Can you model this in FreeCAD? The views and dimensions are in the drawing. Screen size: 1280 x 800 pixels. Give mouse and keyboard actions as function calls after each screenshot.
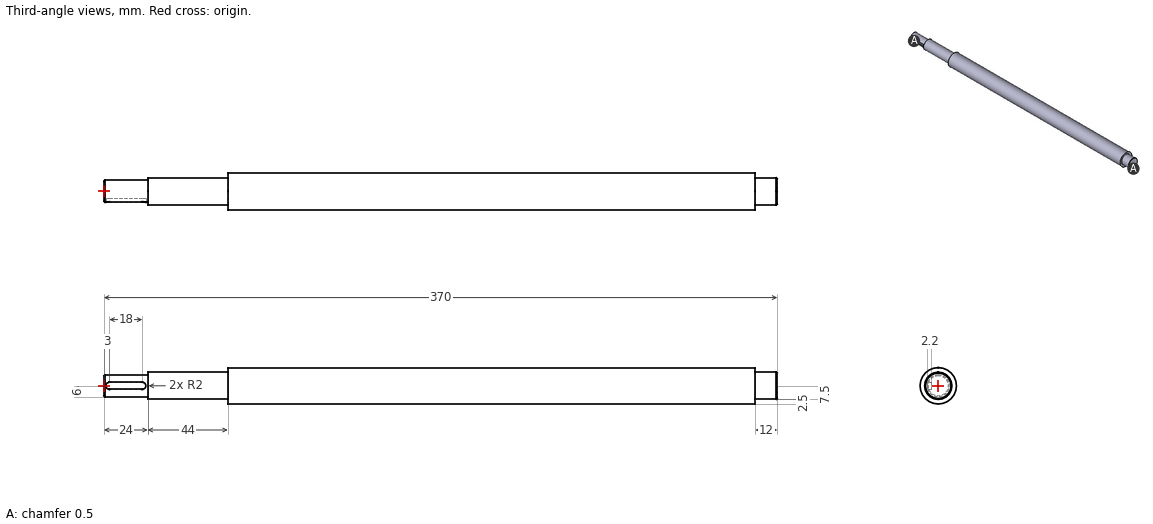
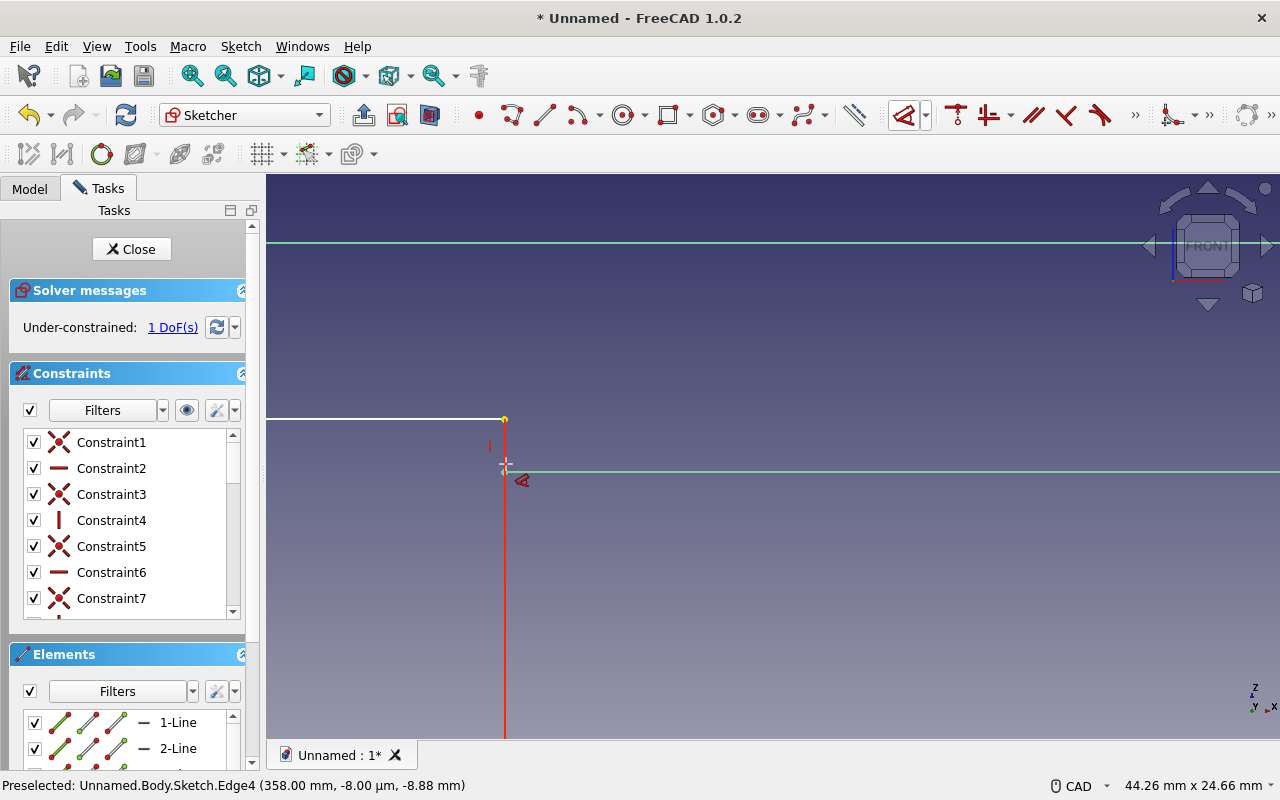
click(505, 456)
click(471, 446)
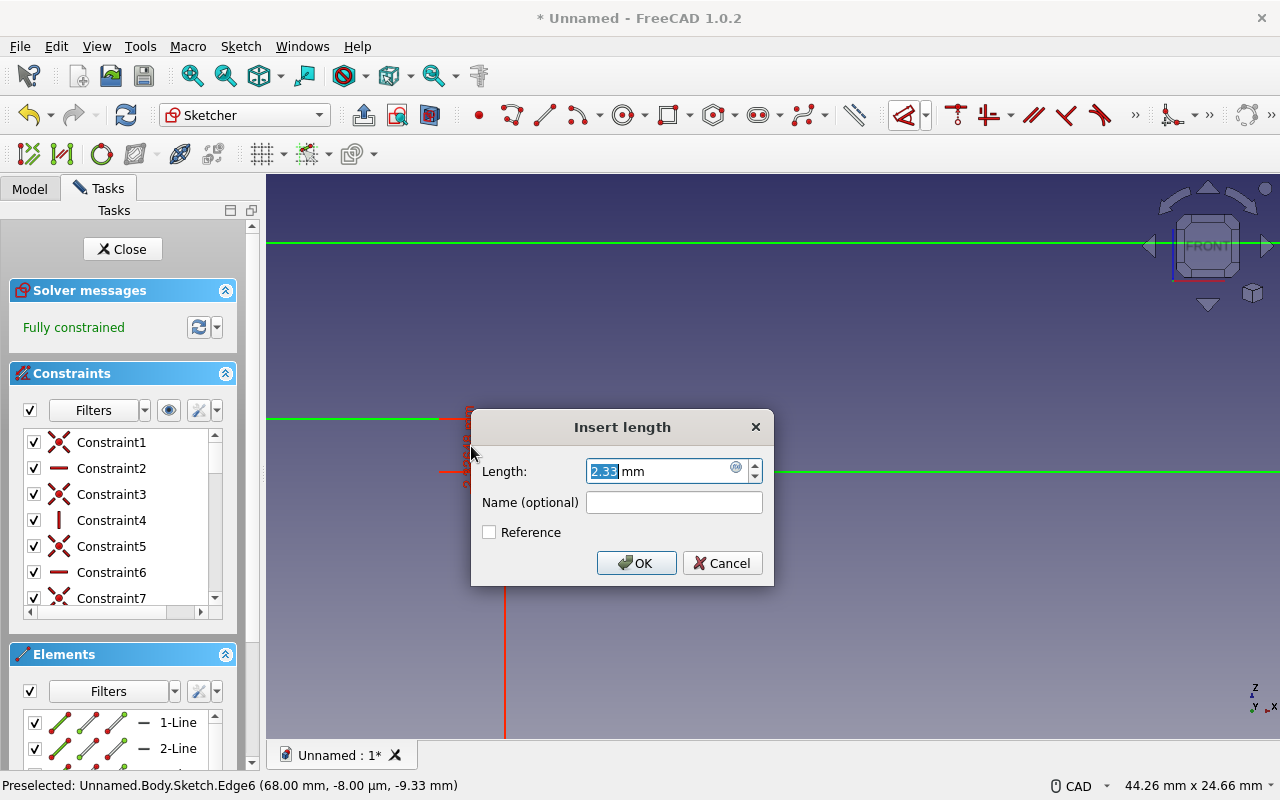
text(2.5)
key(Return)
key(Escape)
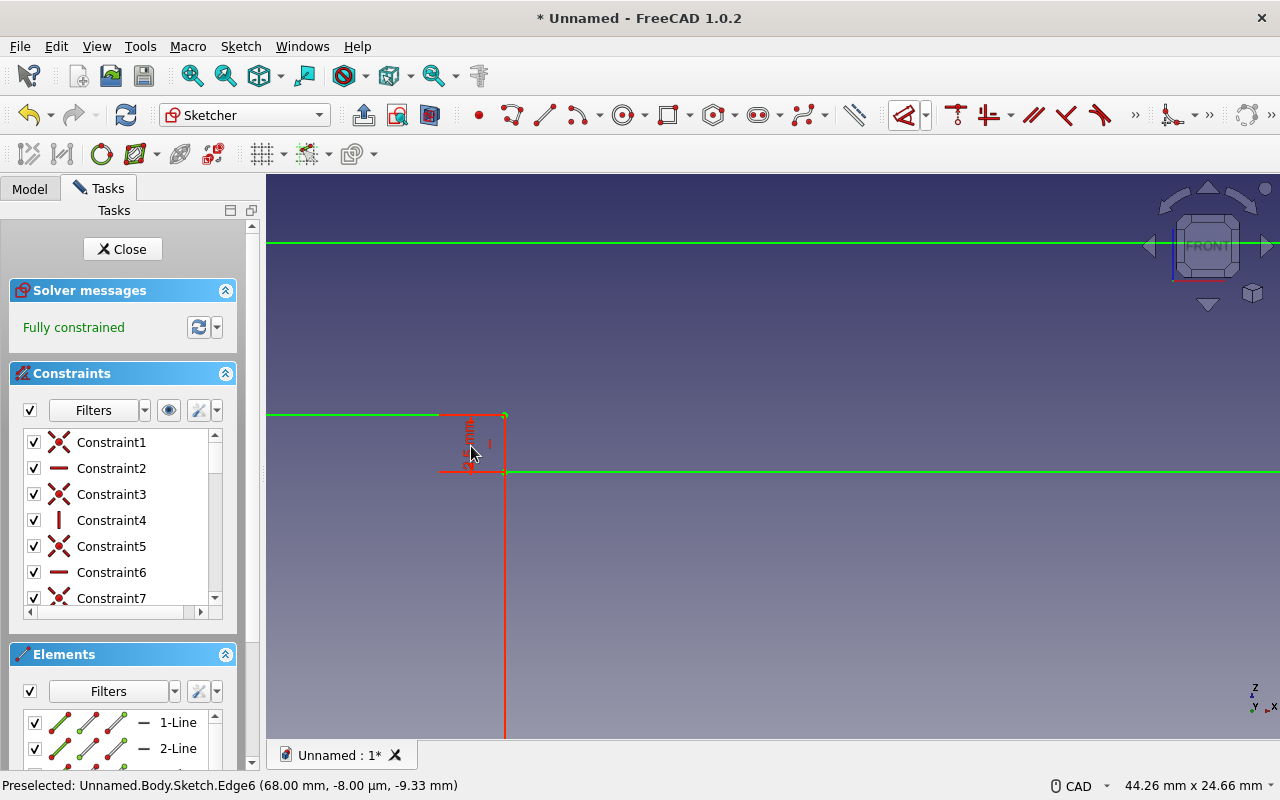
click(123, 249)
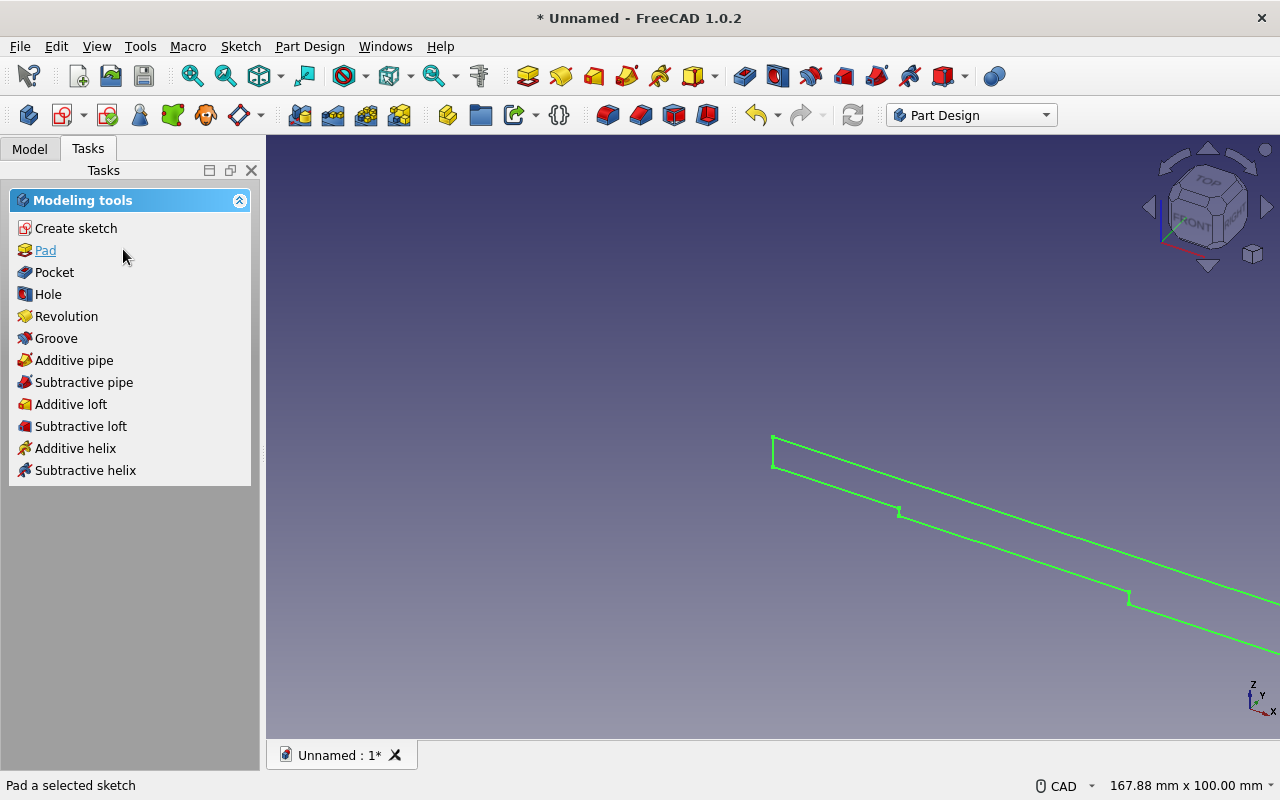
click(561, 76)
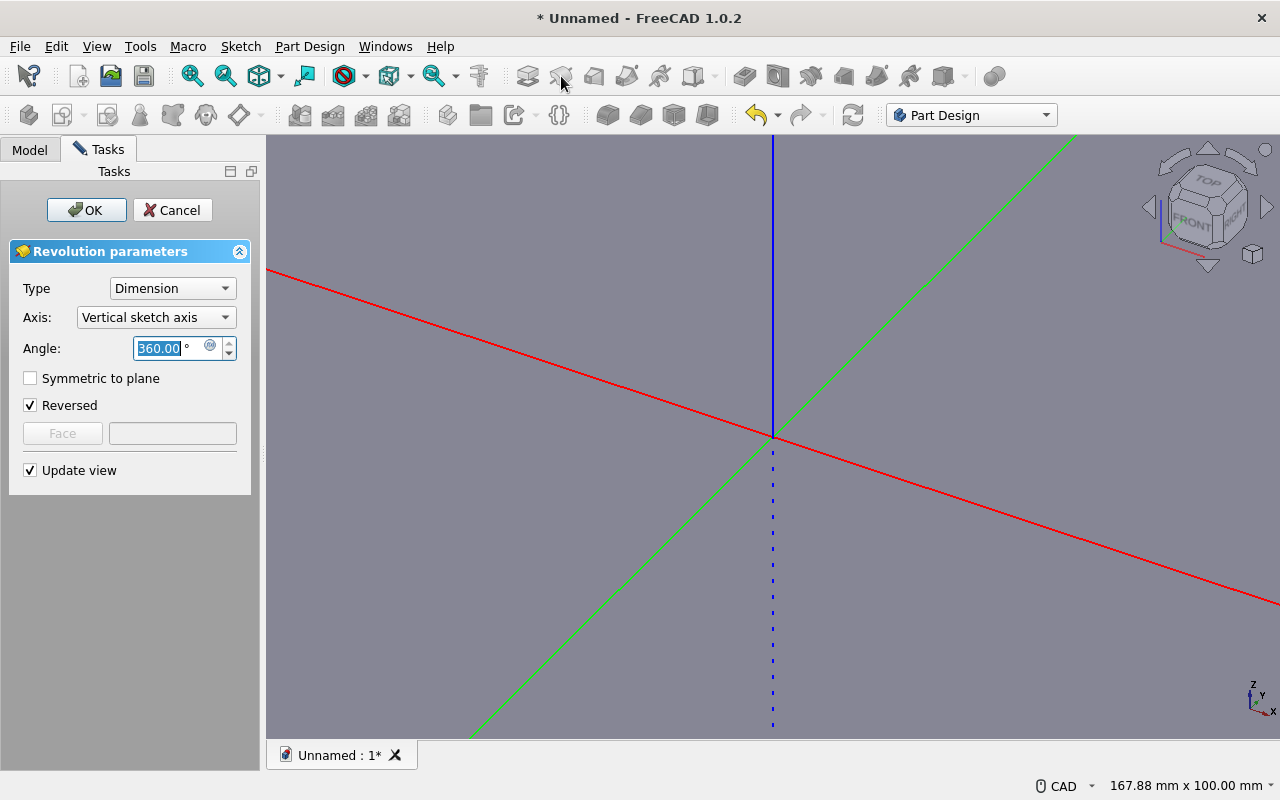
click(157, 318)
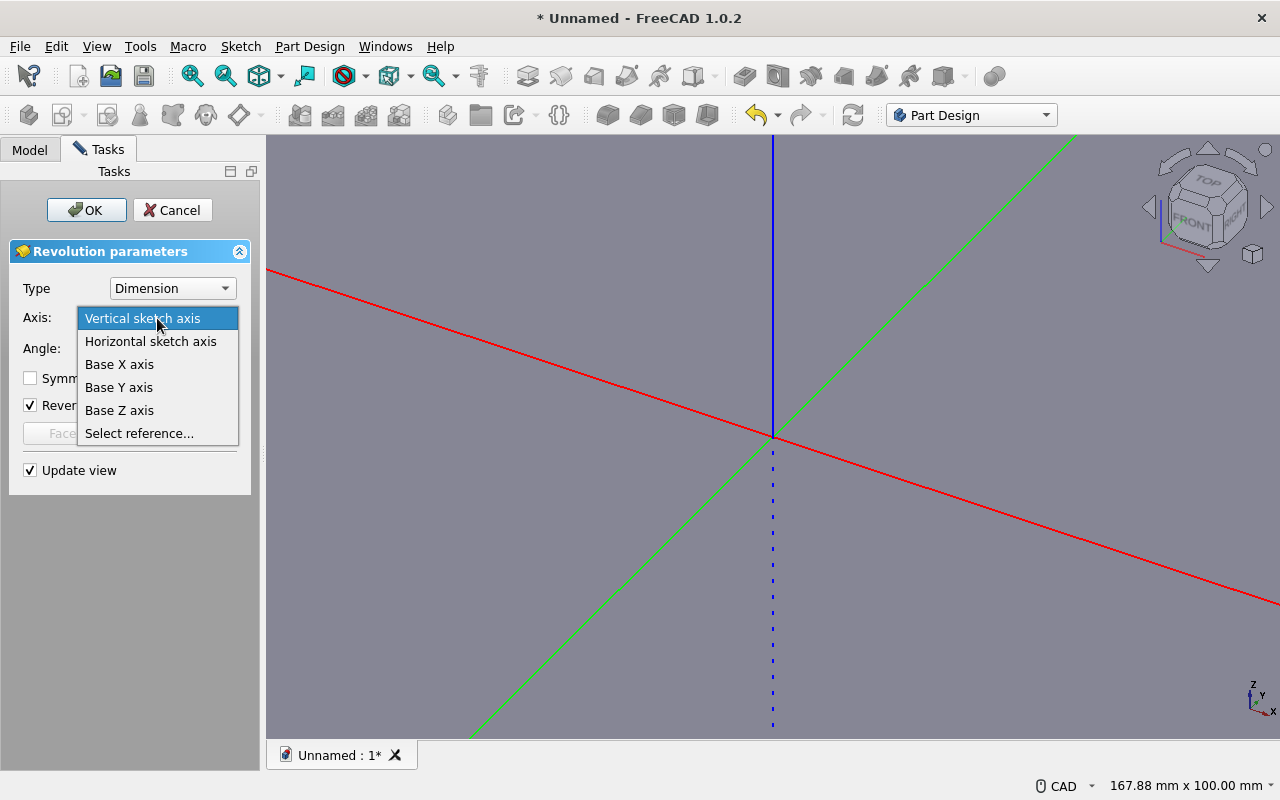
click(156, 342)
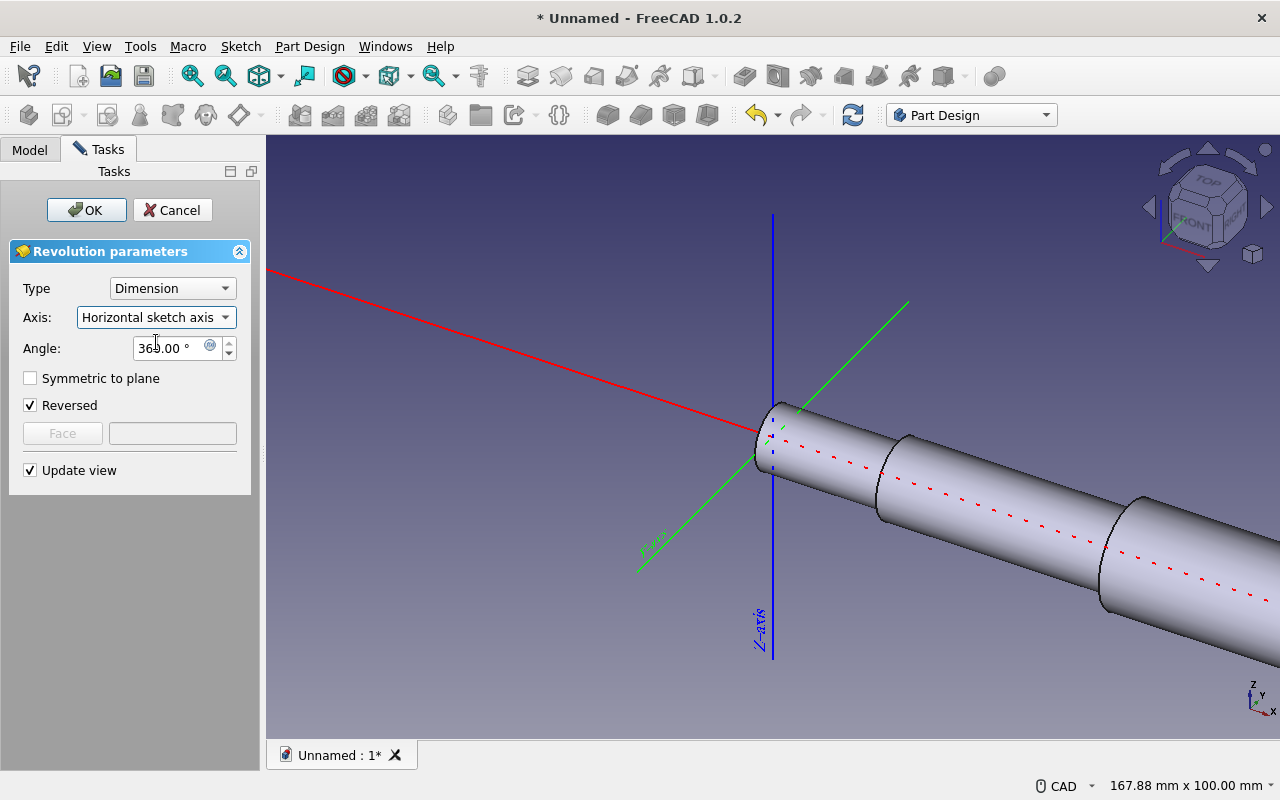
click(87, 210)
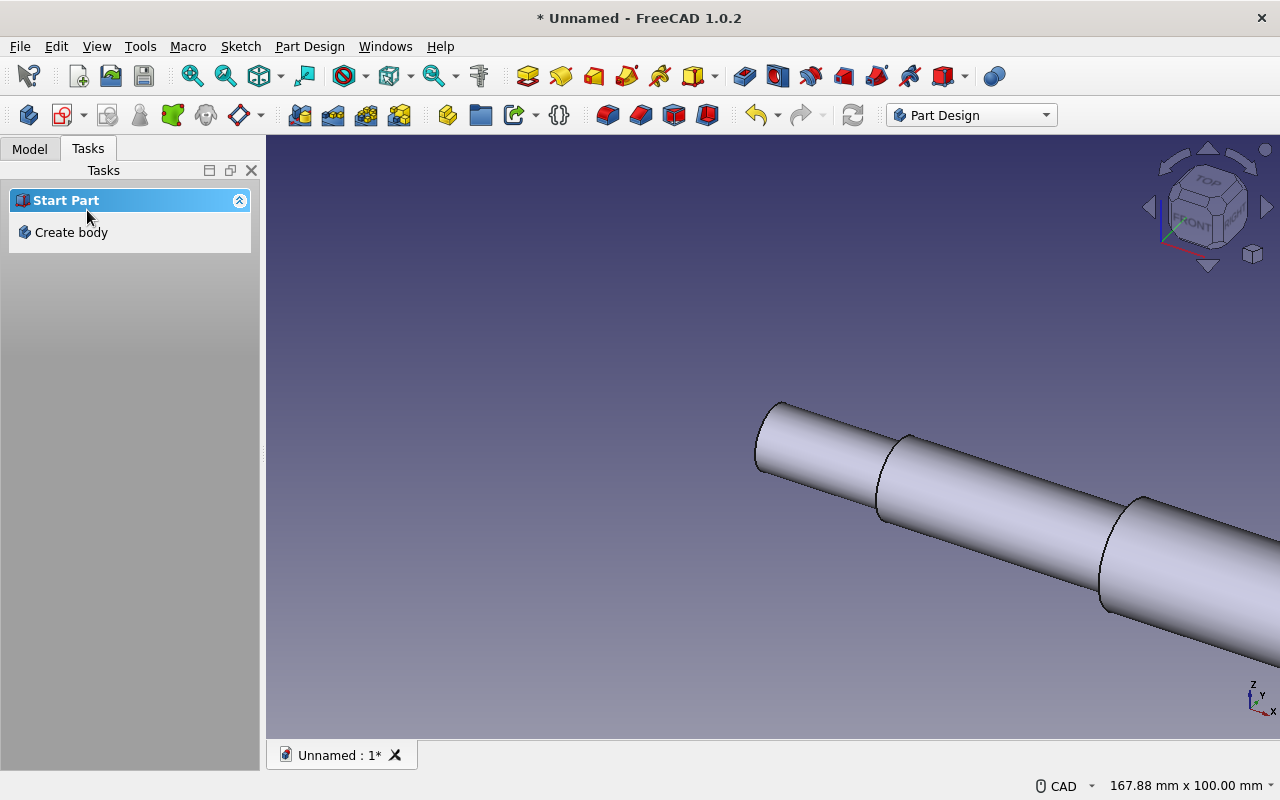
key(v)
key(f)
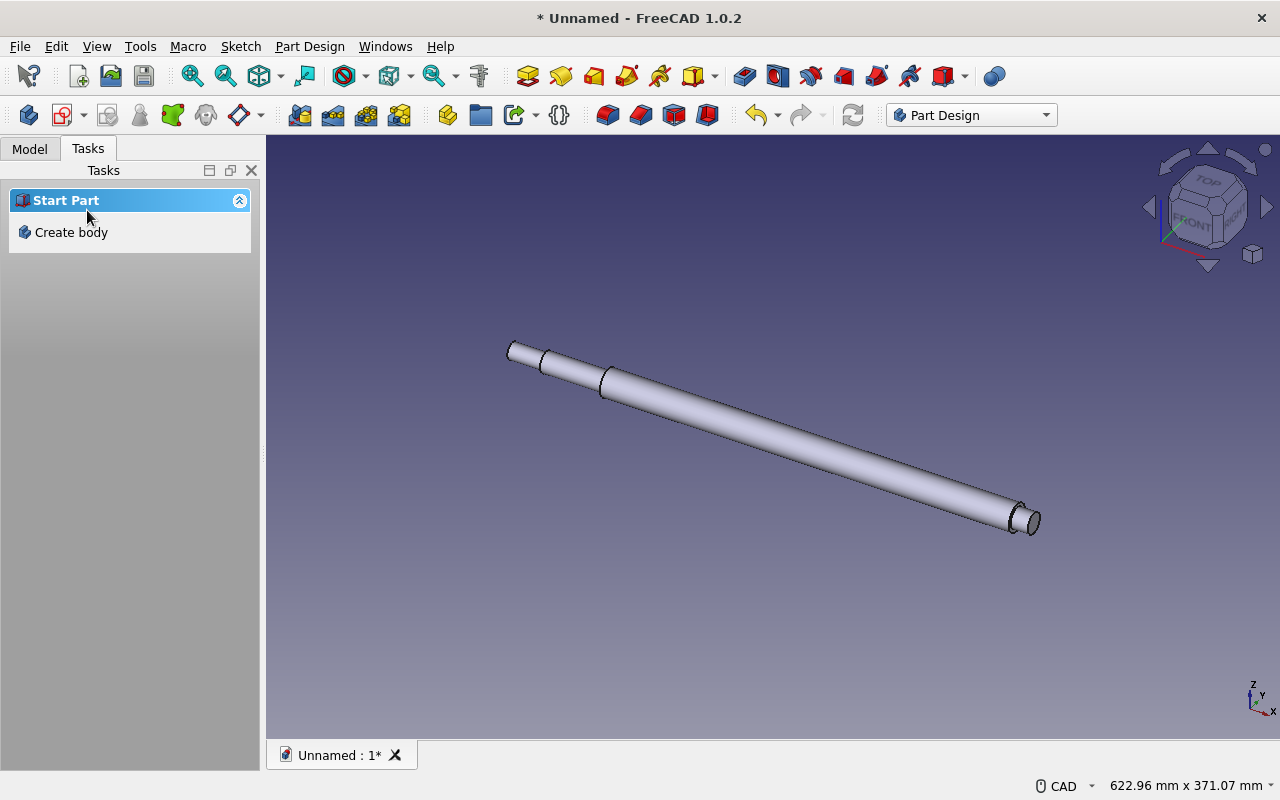
click(30, 148)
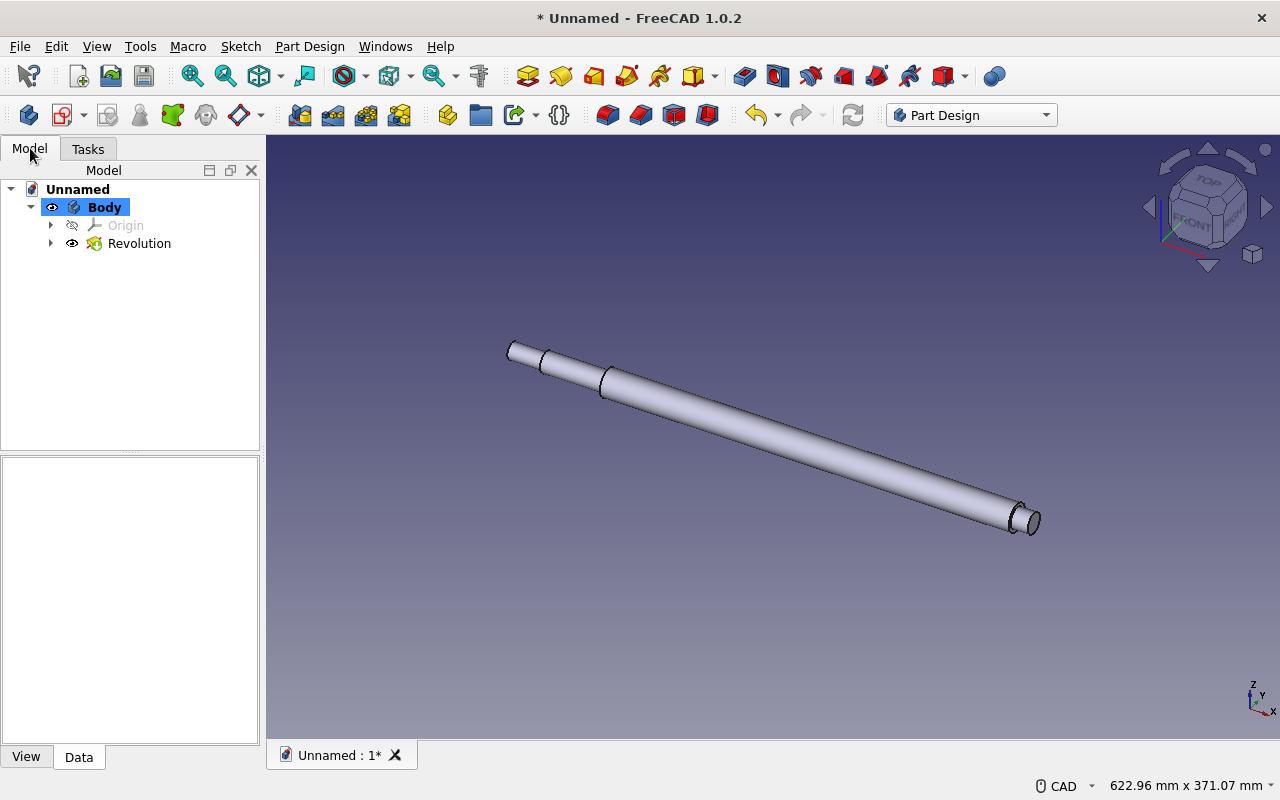
click(51, 225)